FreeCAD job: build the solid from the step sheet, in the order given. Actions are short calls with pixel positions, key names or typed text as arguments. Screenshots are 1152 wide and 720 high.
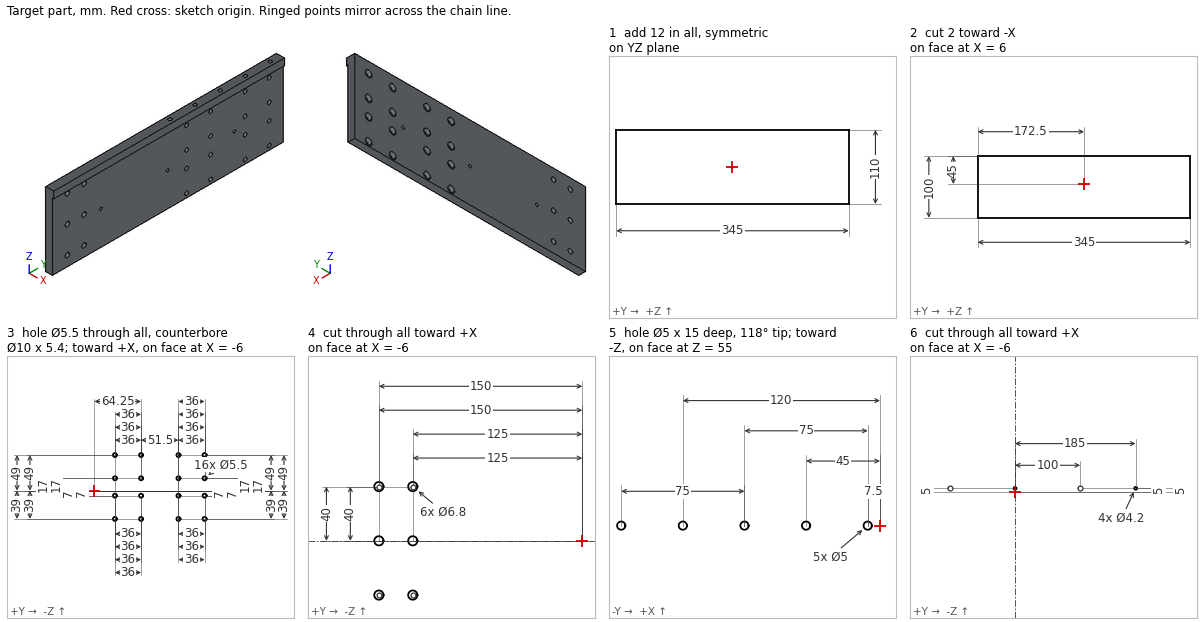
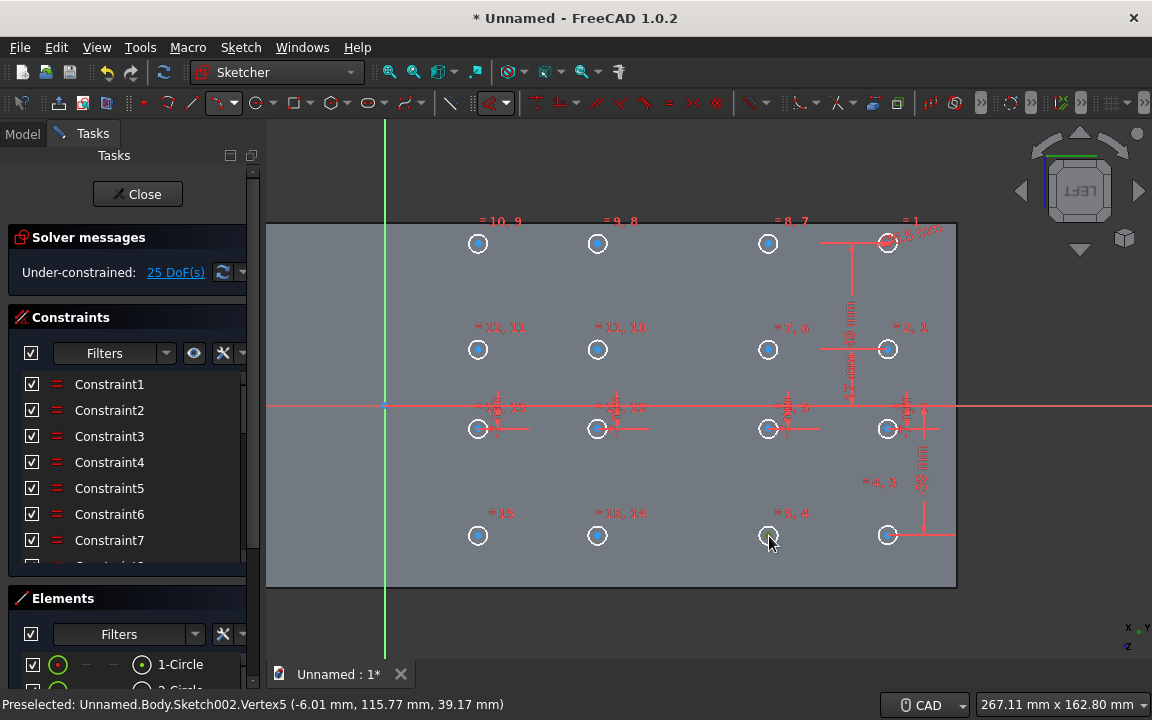
click(508, 104)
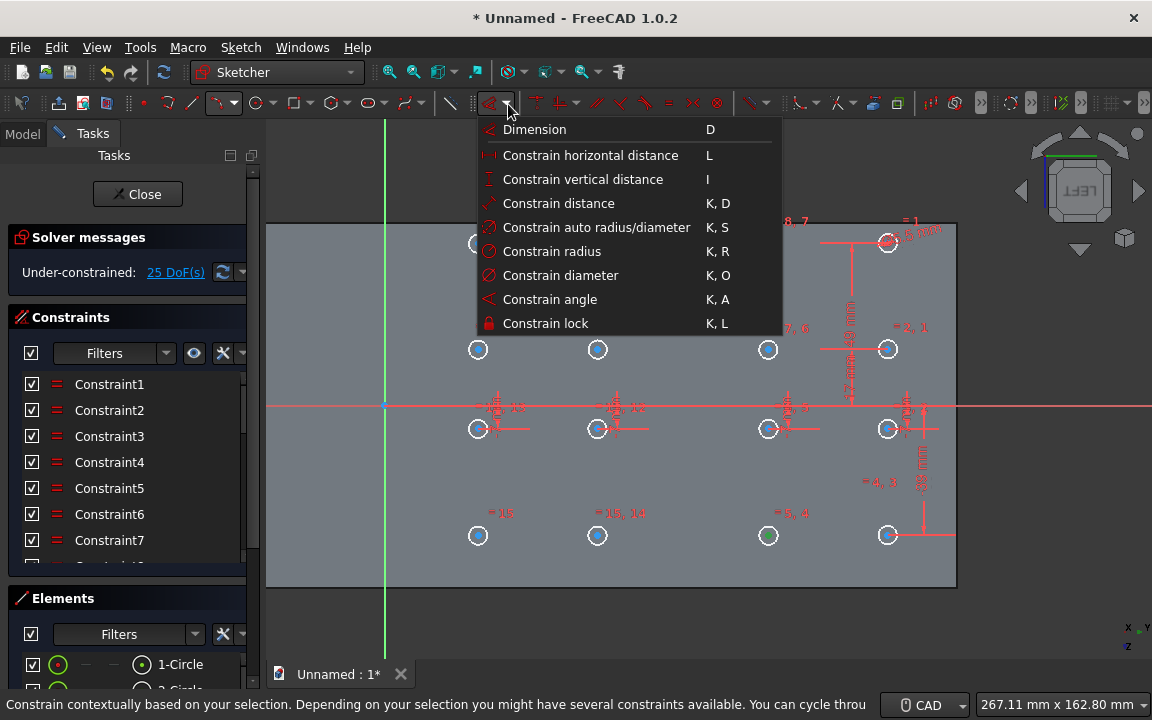
click(630, 179)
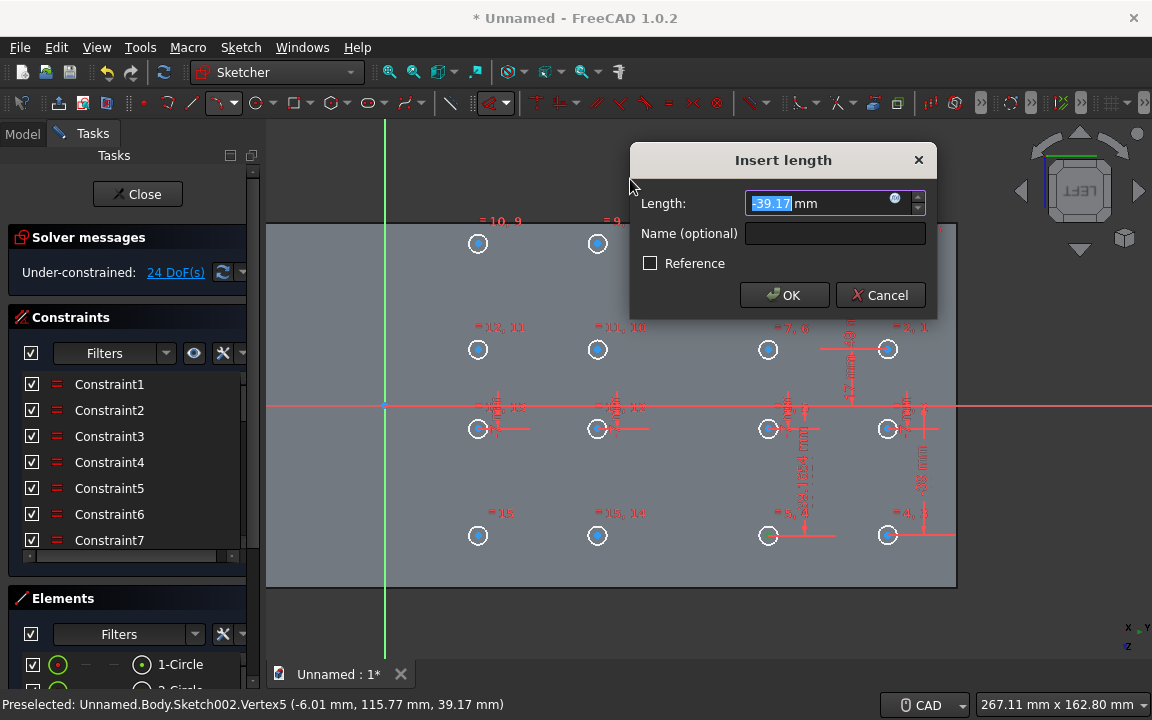
text(-39)
key(Return)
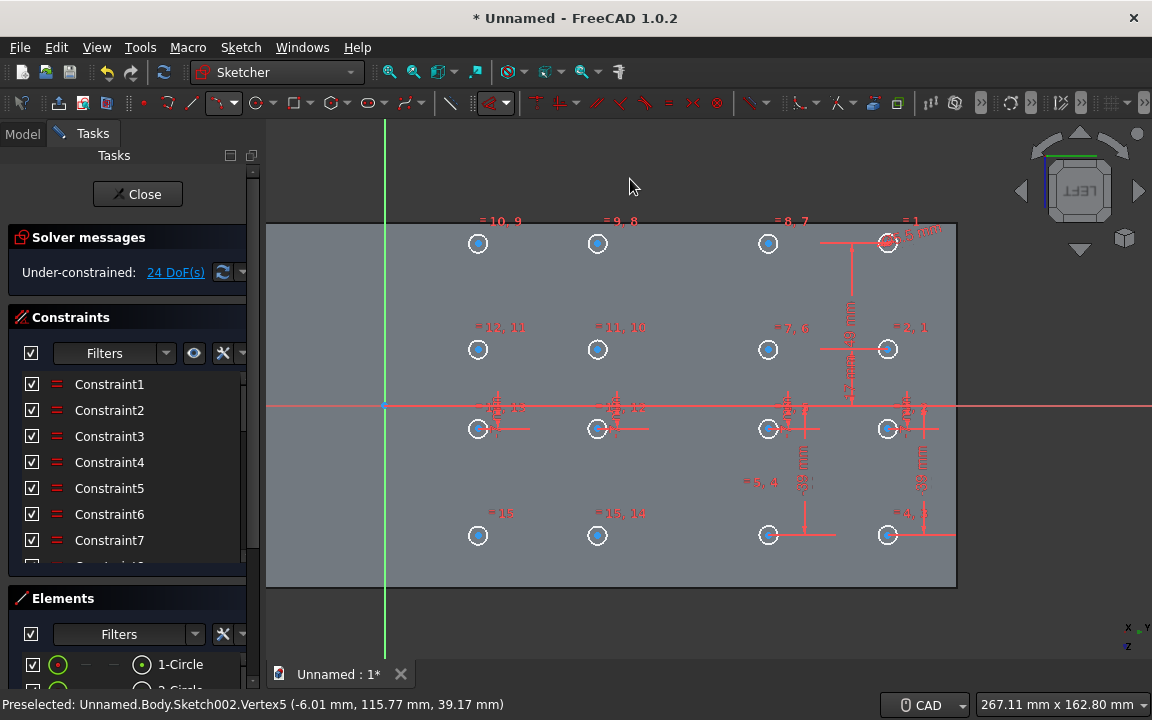
click(768, 350)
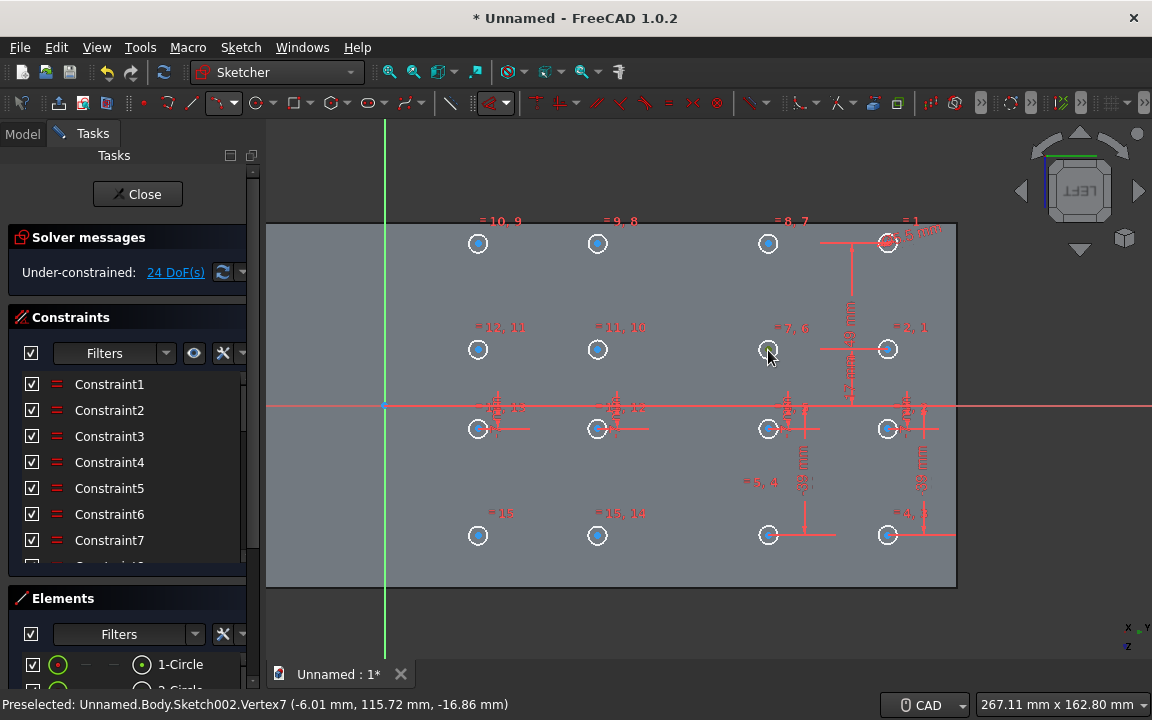
click(508, 104)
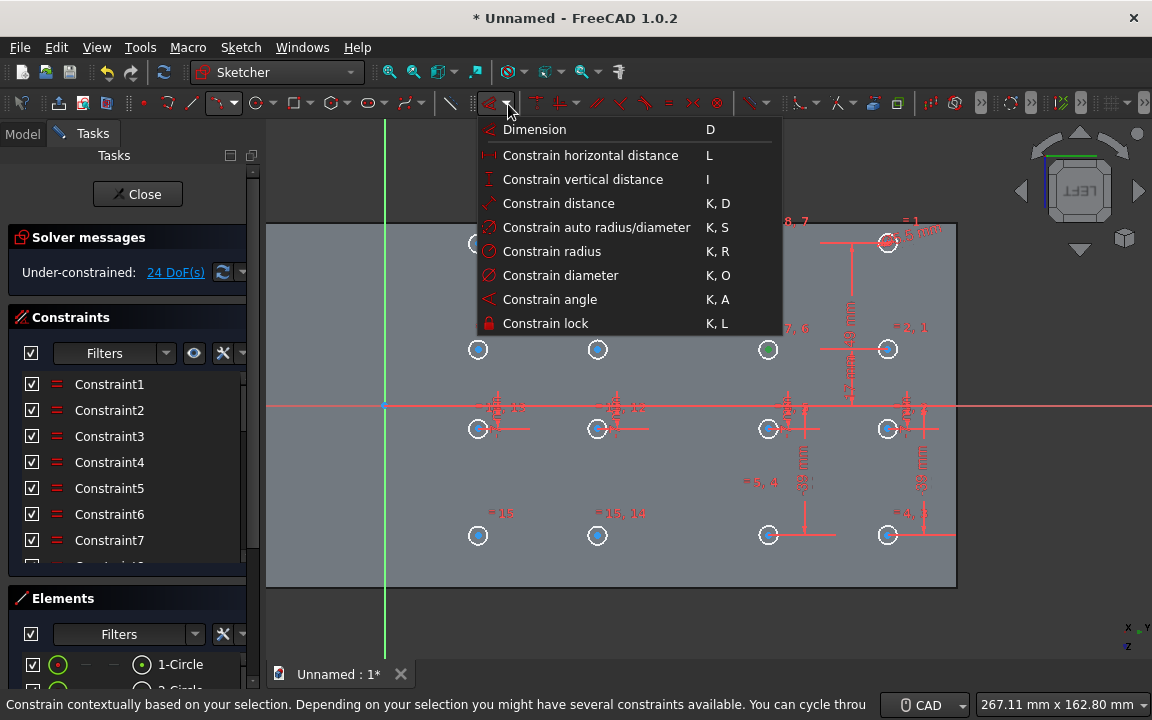
click(630, 179)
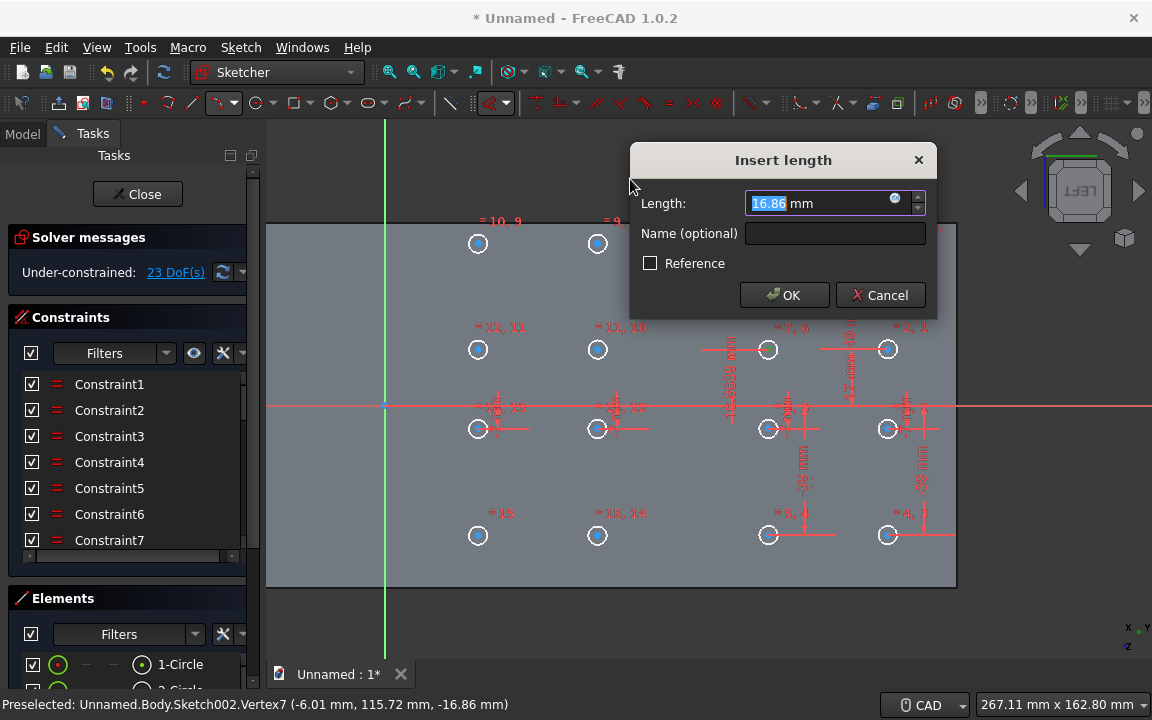
text(17)
key(Return)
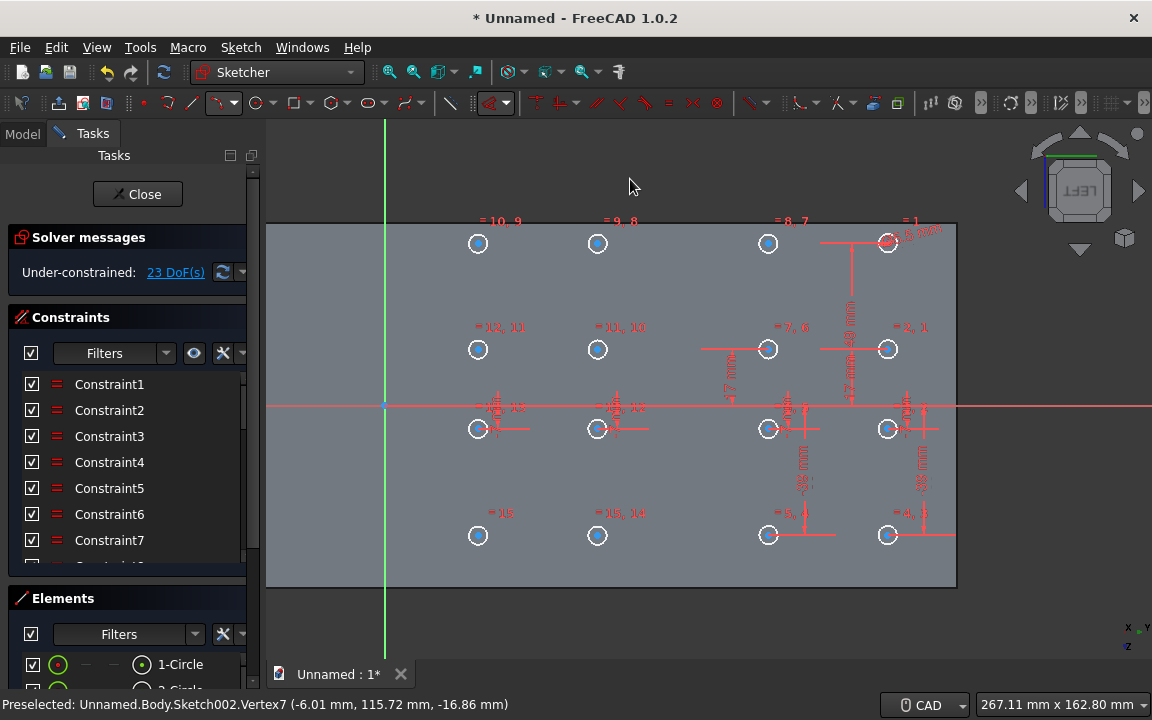
click(768, 244)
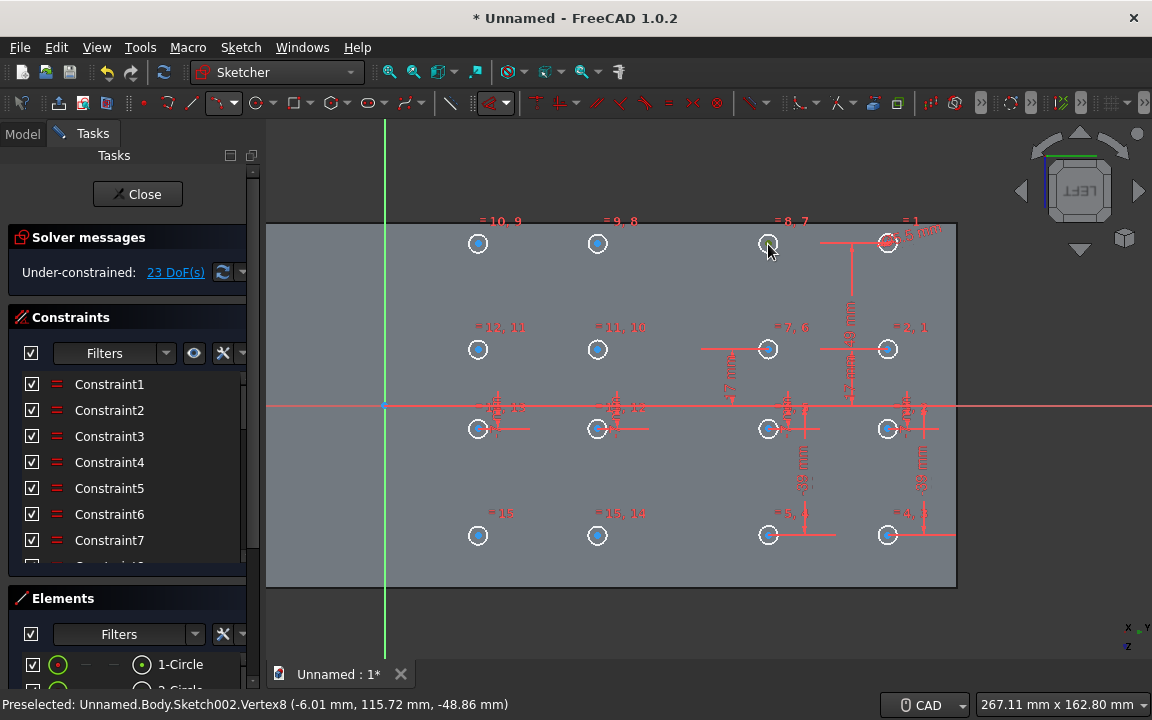
key(i)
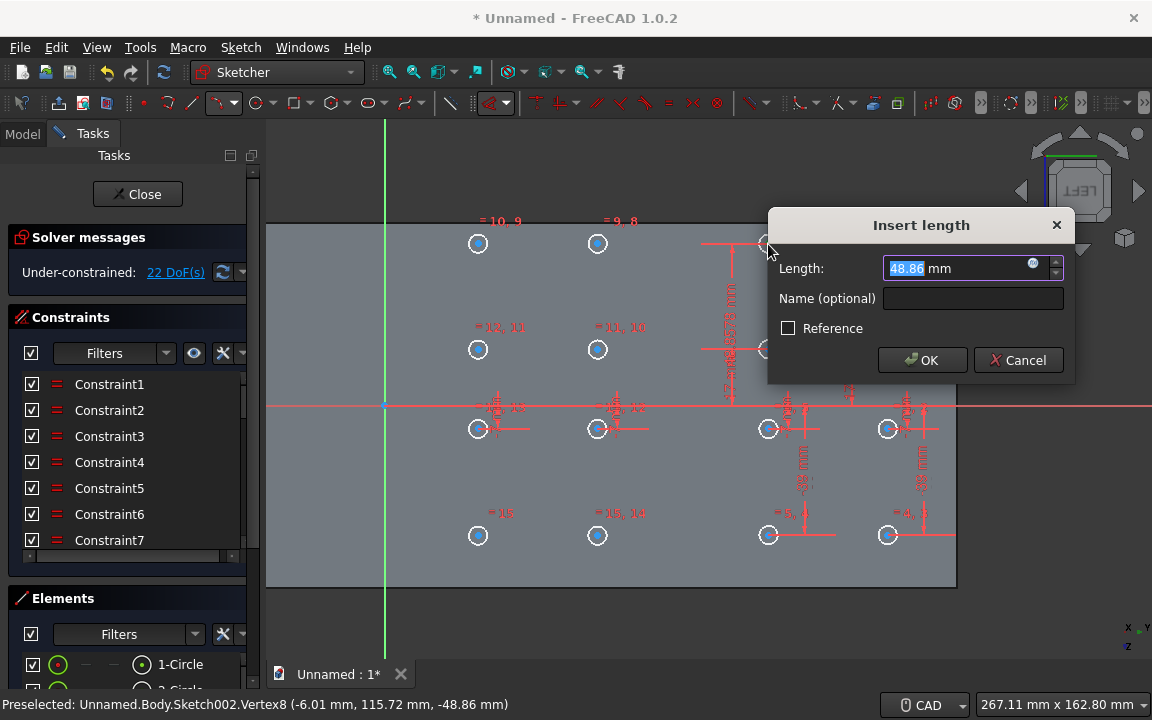
text(49)
key(Return)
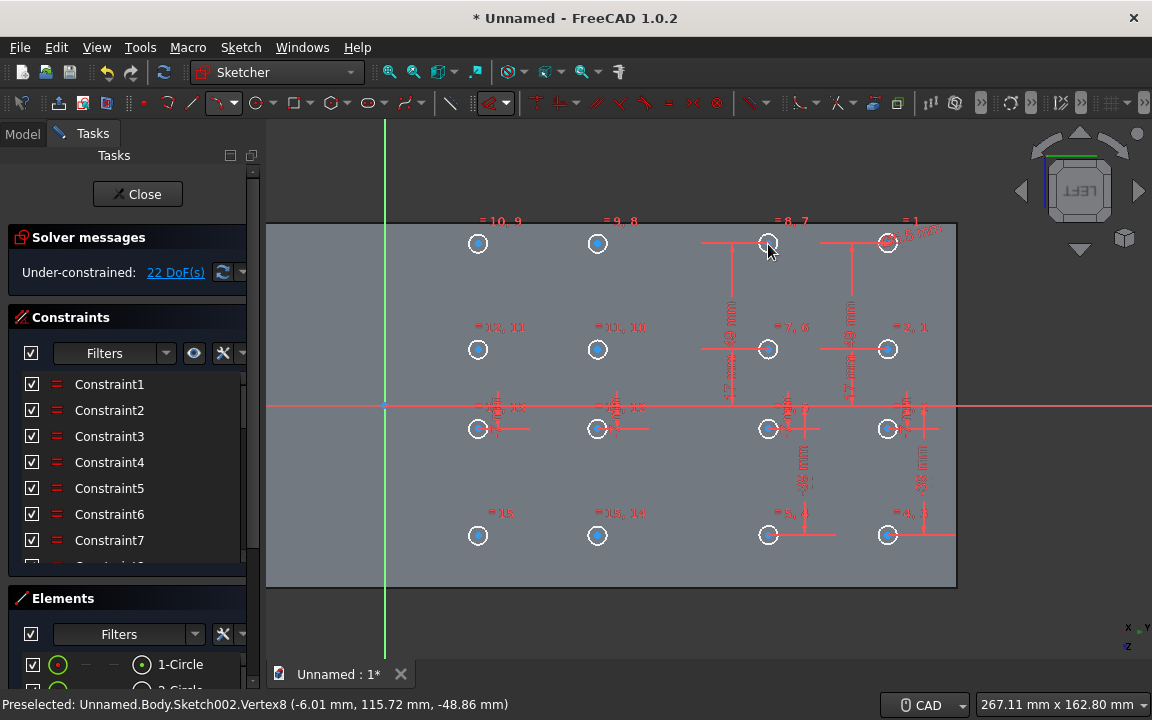
click(598, 244)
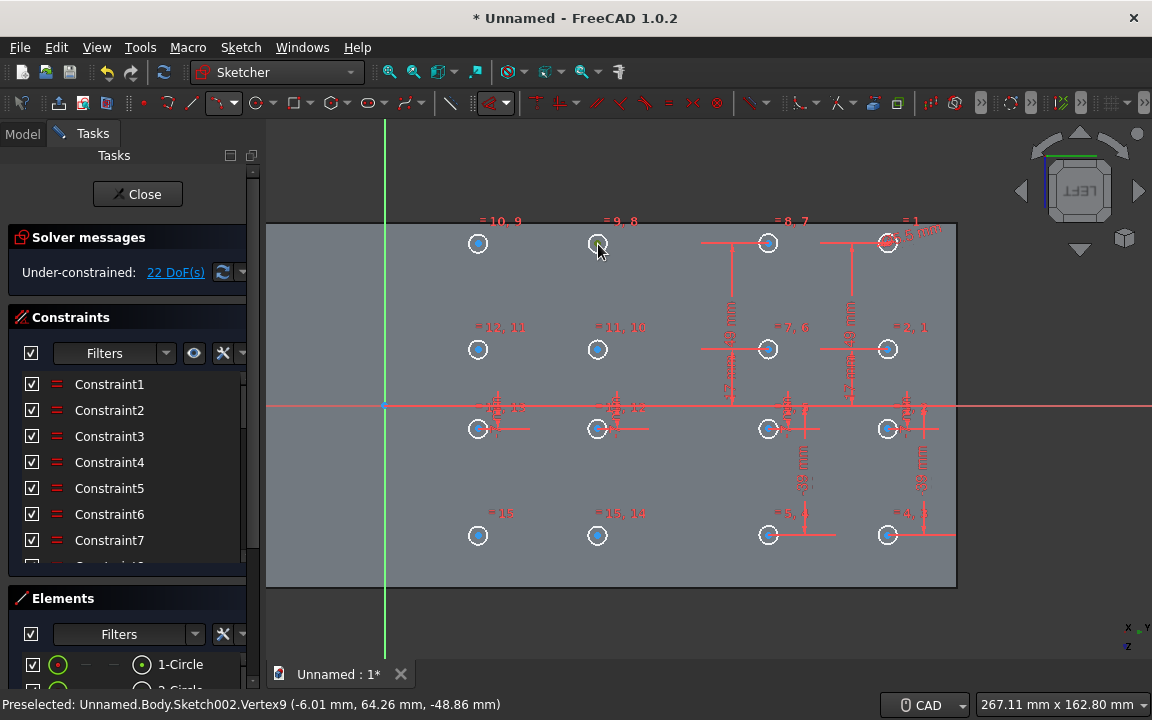
key(i)